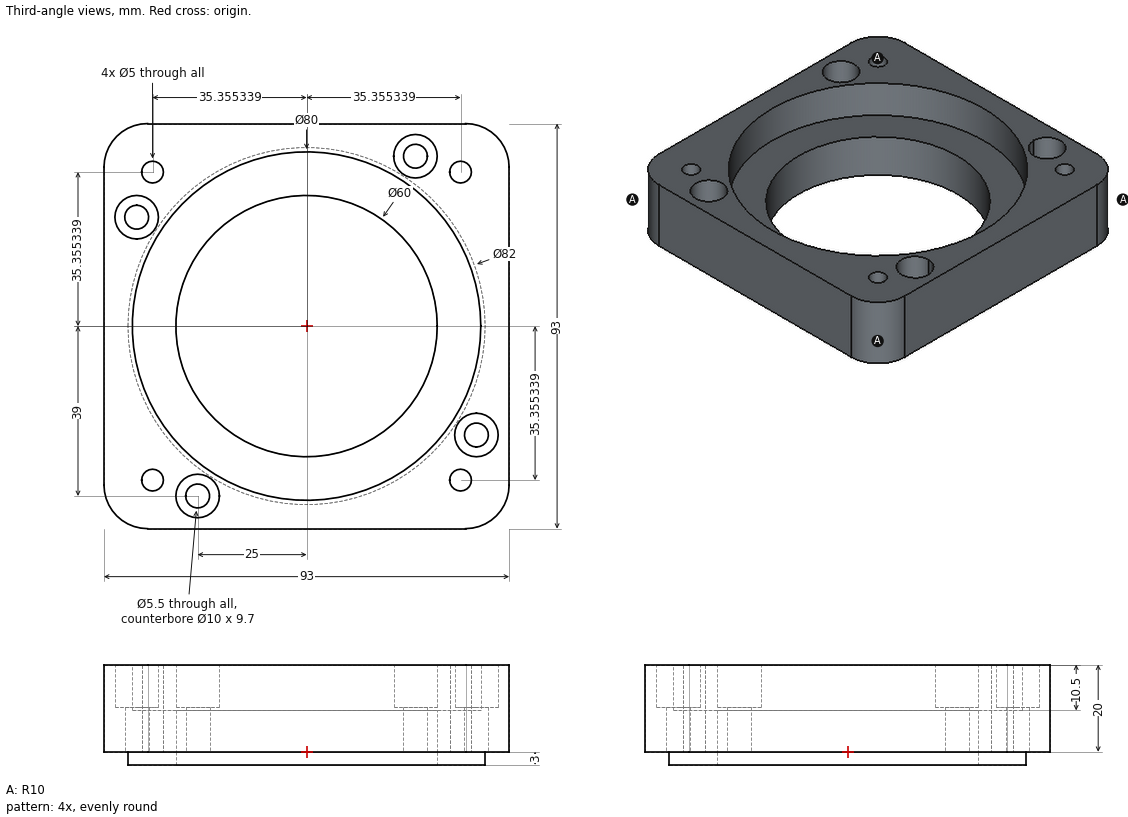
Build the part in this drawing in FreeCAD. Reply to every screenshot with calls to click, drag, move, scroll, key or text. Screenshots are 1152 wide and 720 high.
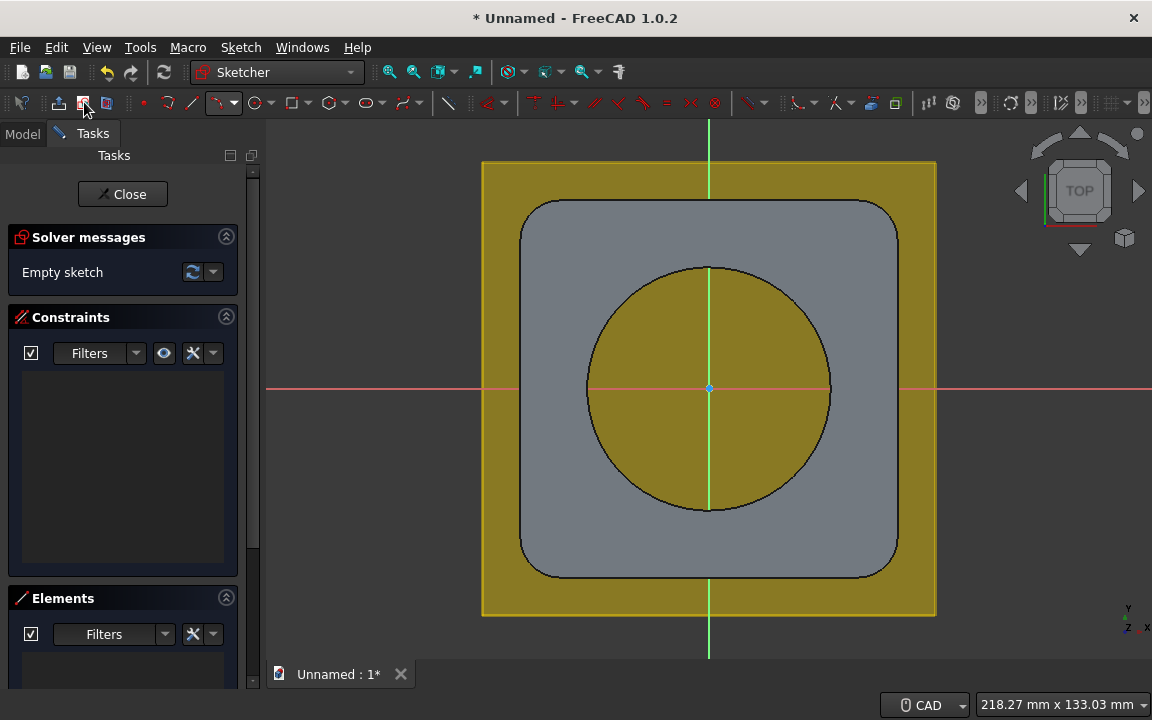
click(108, 104)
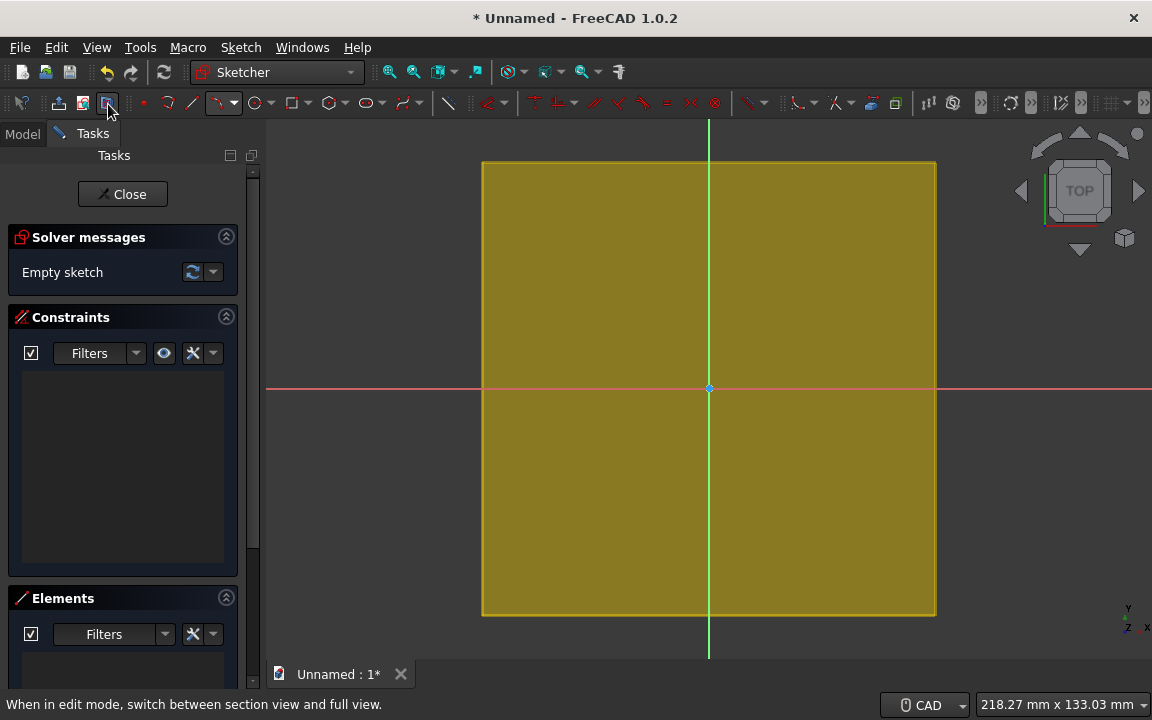
click(256, 104)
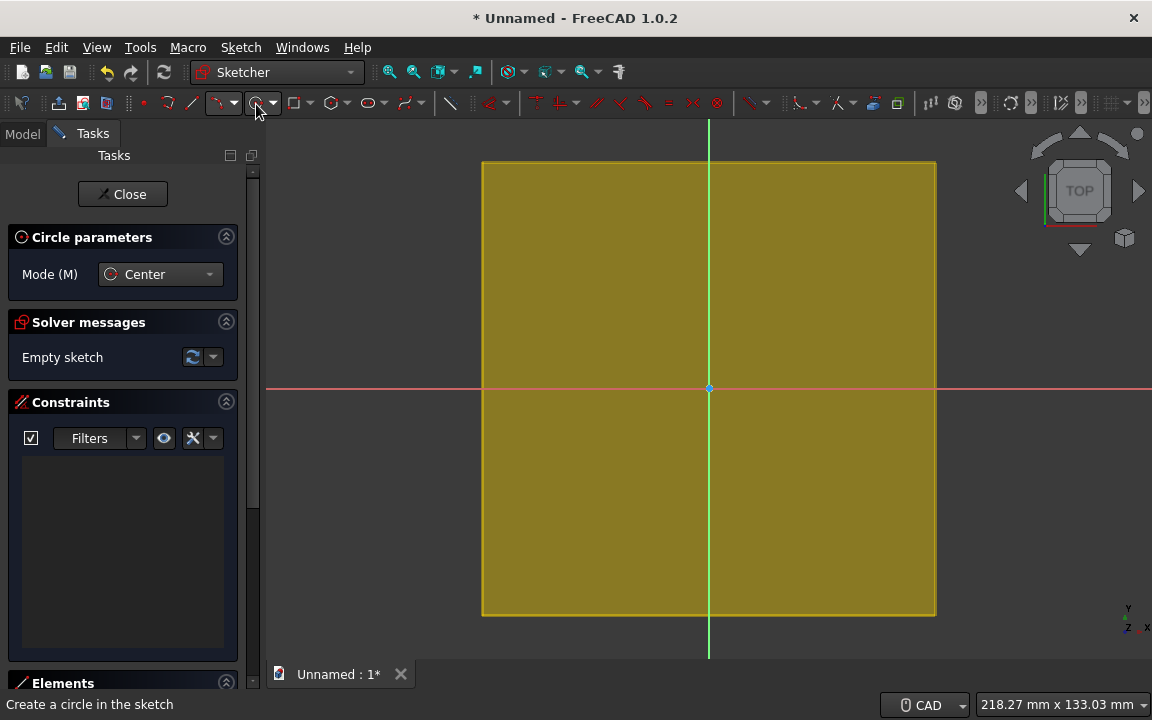
click(709, 389)
click(827, 271)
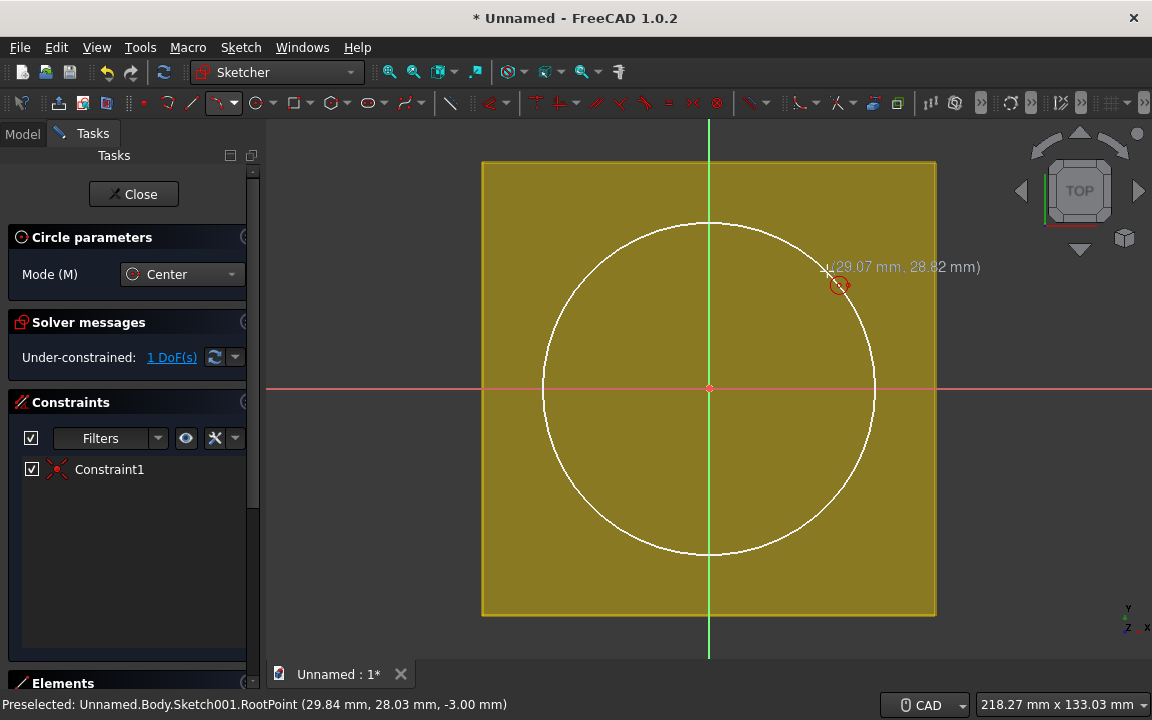
click(709, 389)
click(795, 303)
key(Escape)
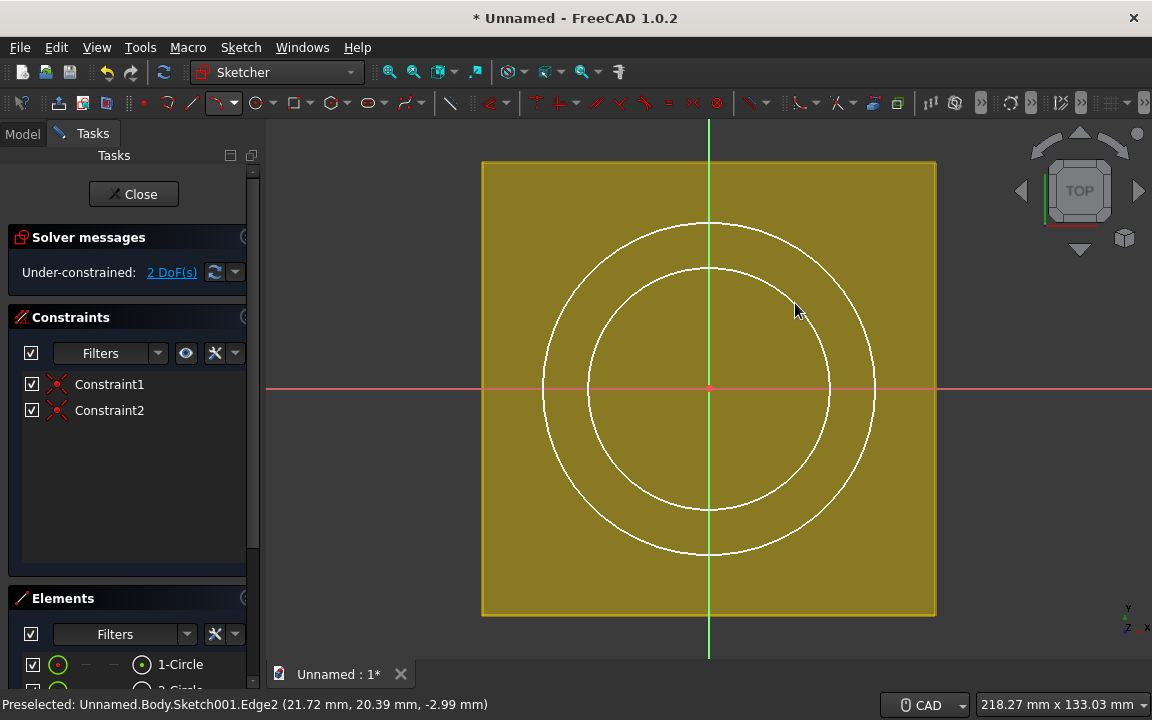
click(490, 104)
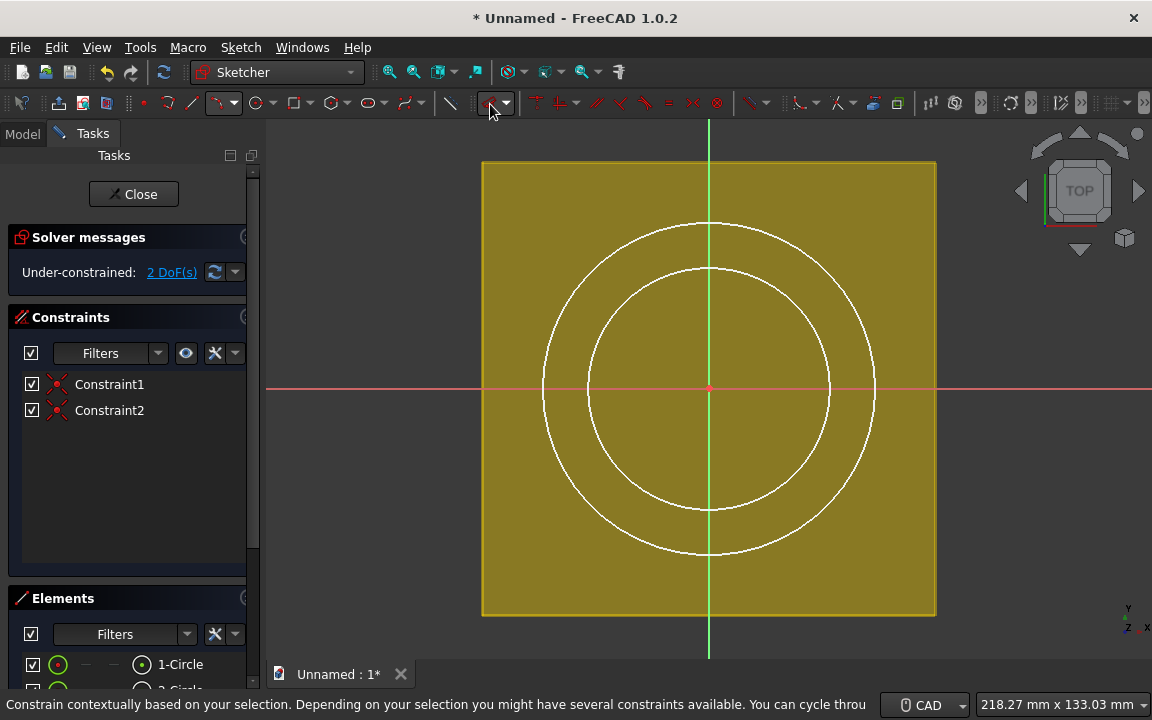
click(826, 271)
click(849, 248)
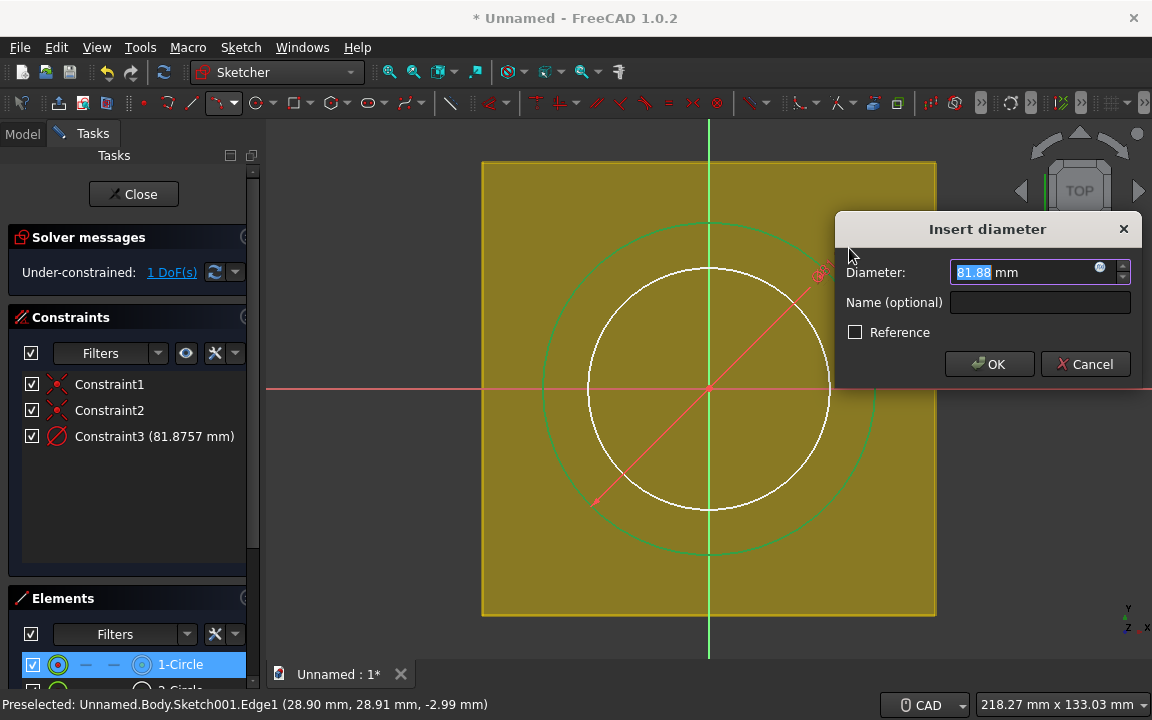
text(82)
key(Return)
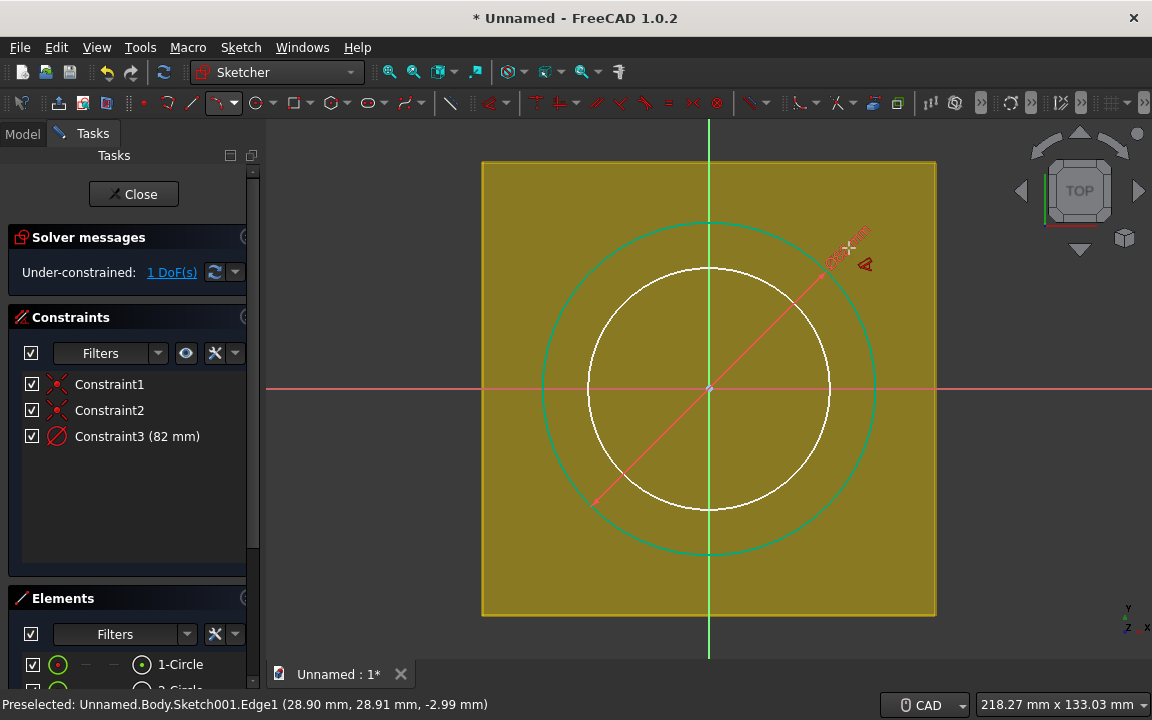
click(794, 303)
click(816, 280)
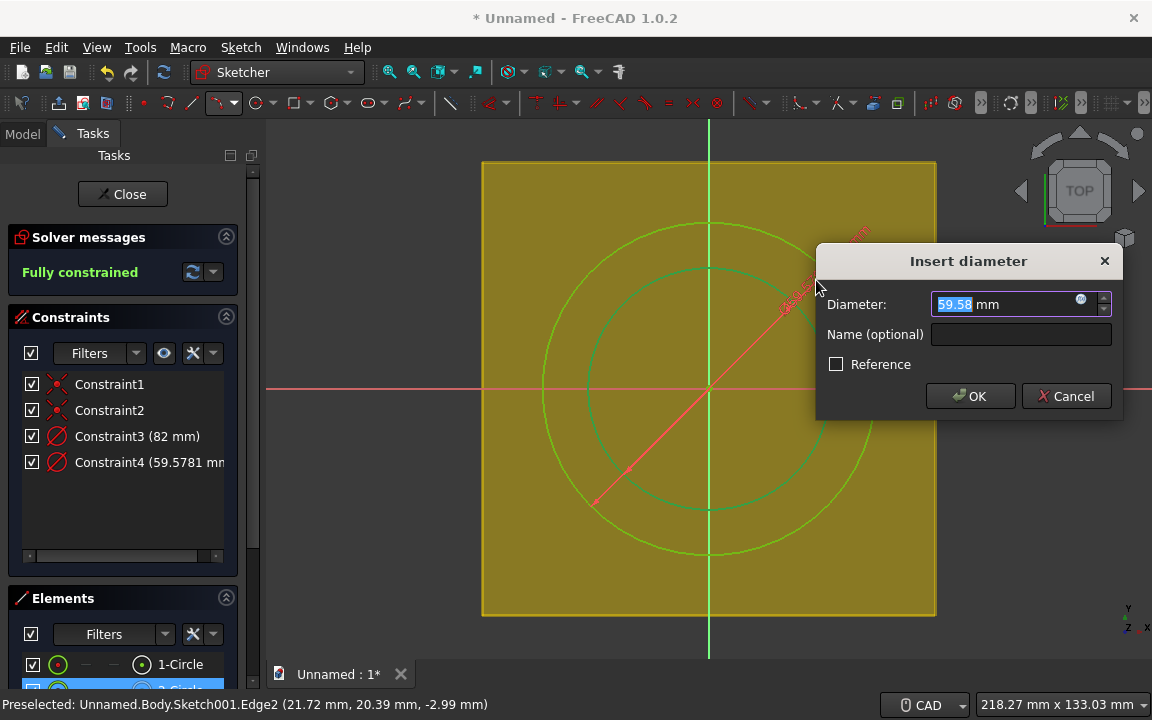
text(60)
key(Return)
key(Escape)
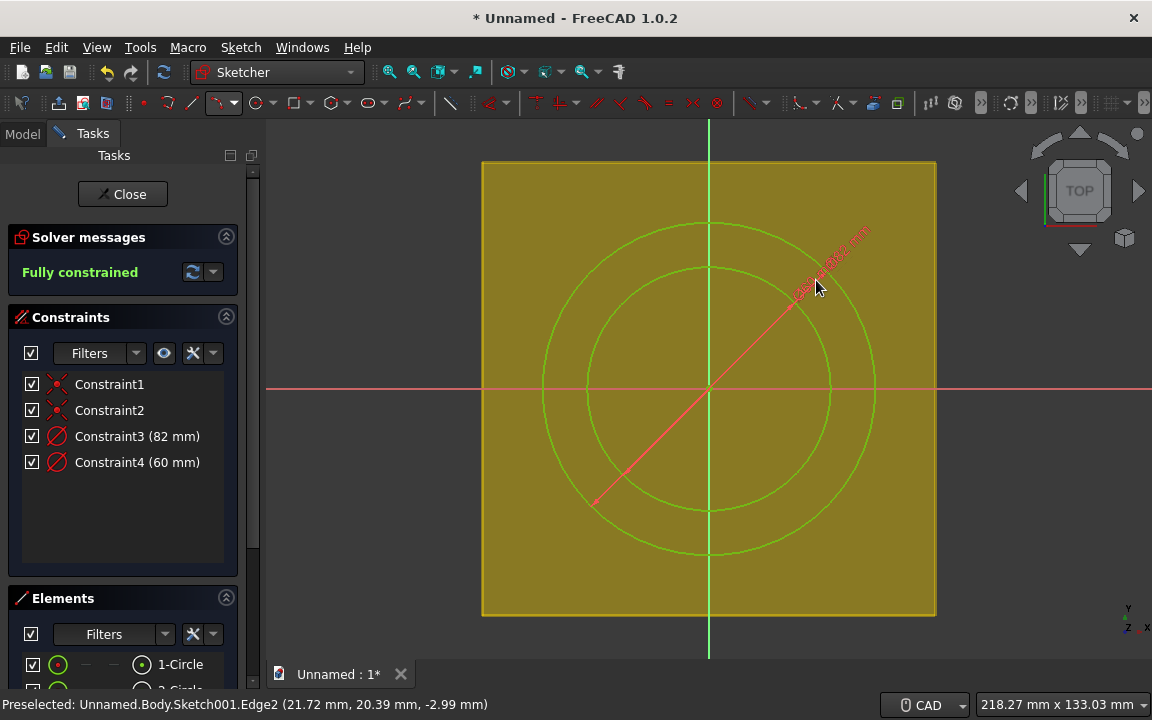
click(123, 194)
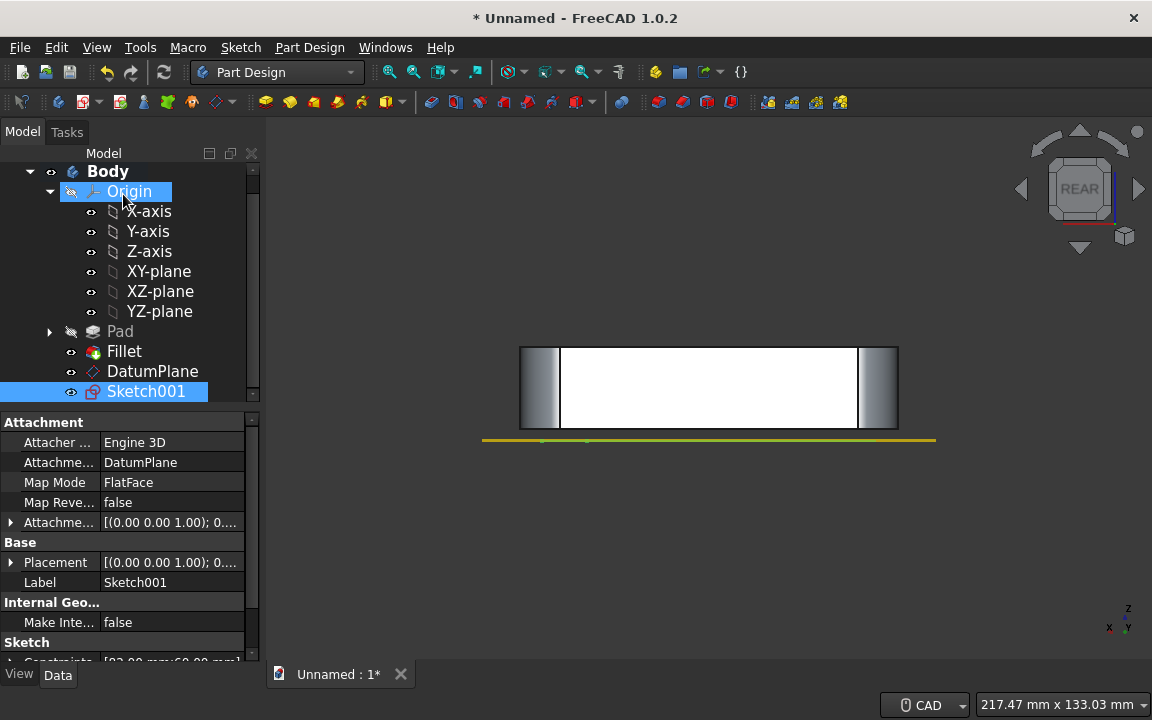
click(266, 102)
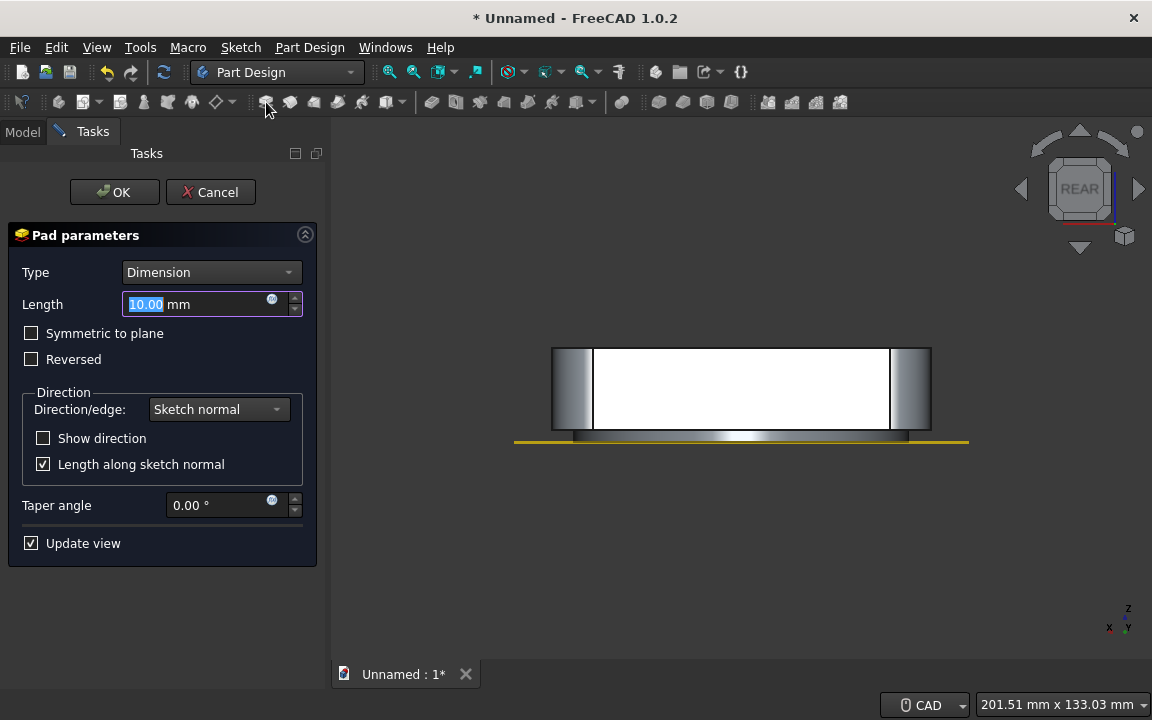
text(3)
key(Tab)